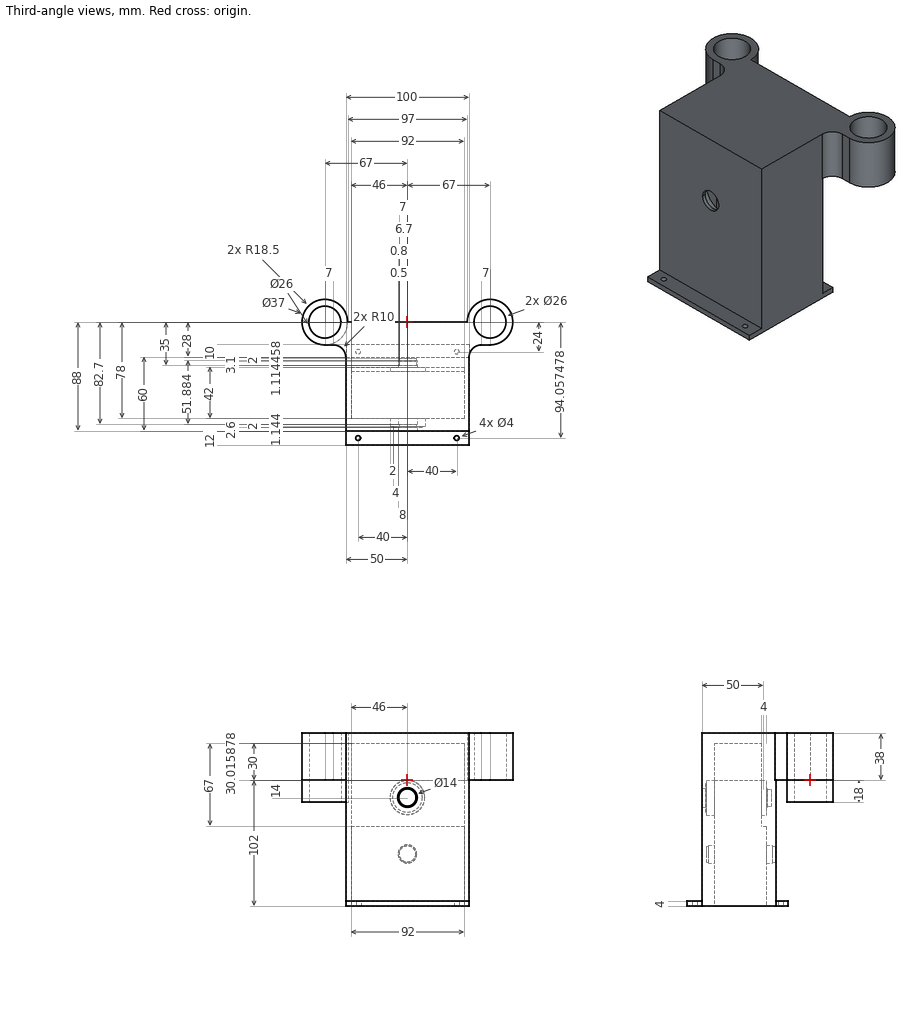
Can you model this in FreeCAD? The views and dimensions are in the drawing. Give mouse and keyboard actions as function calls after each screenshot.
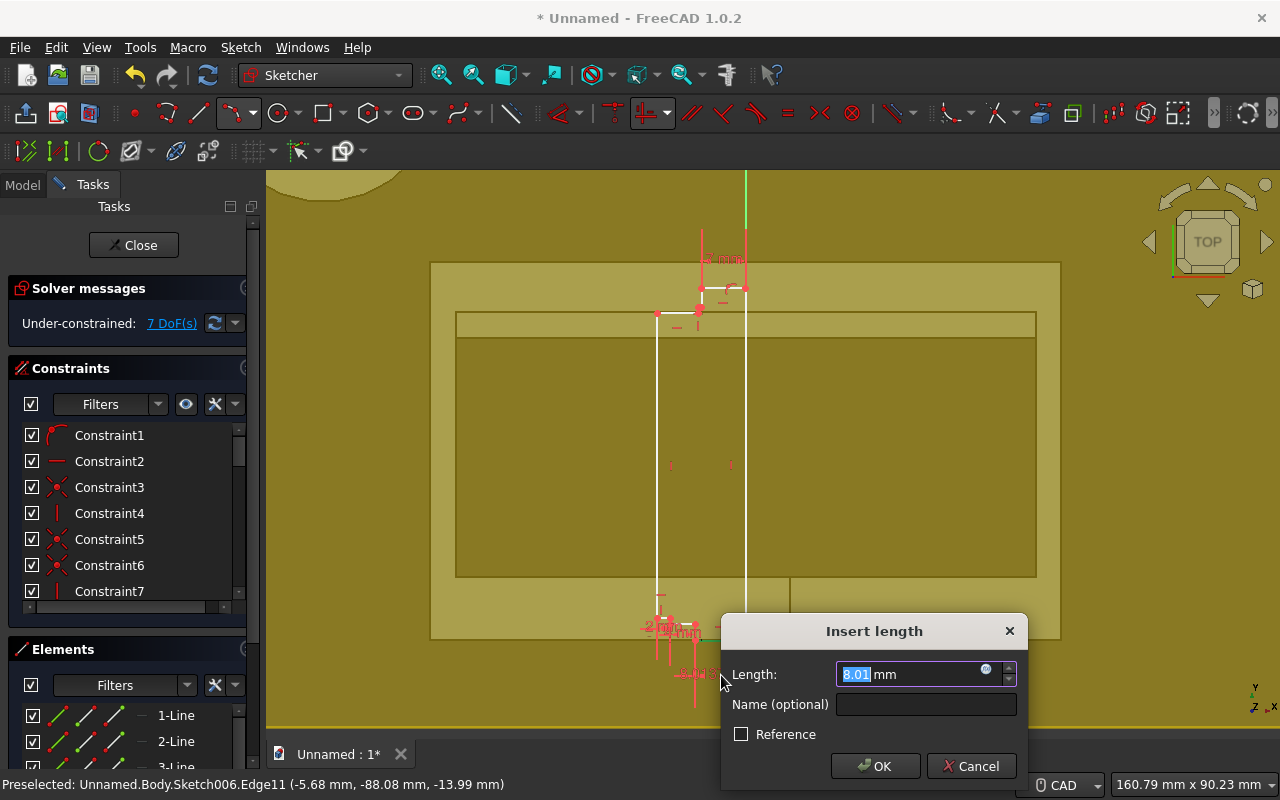
text(8)
key(Return)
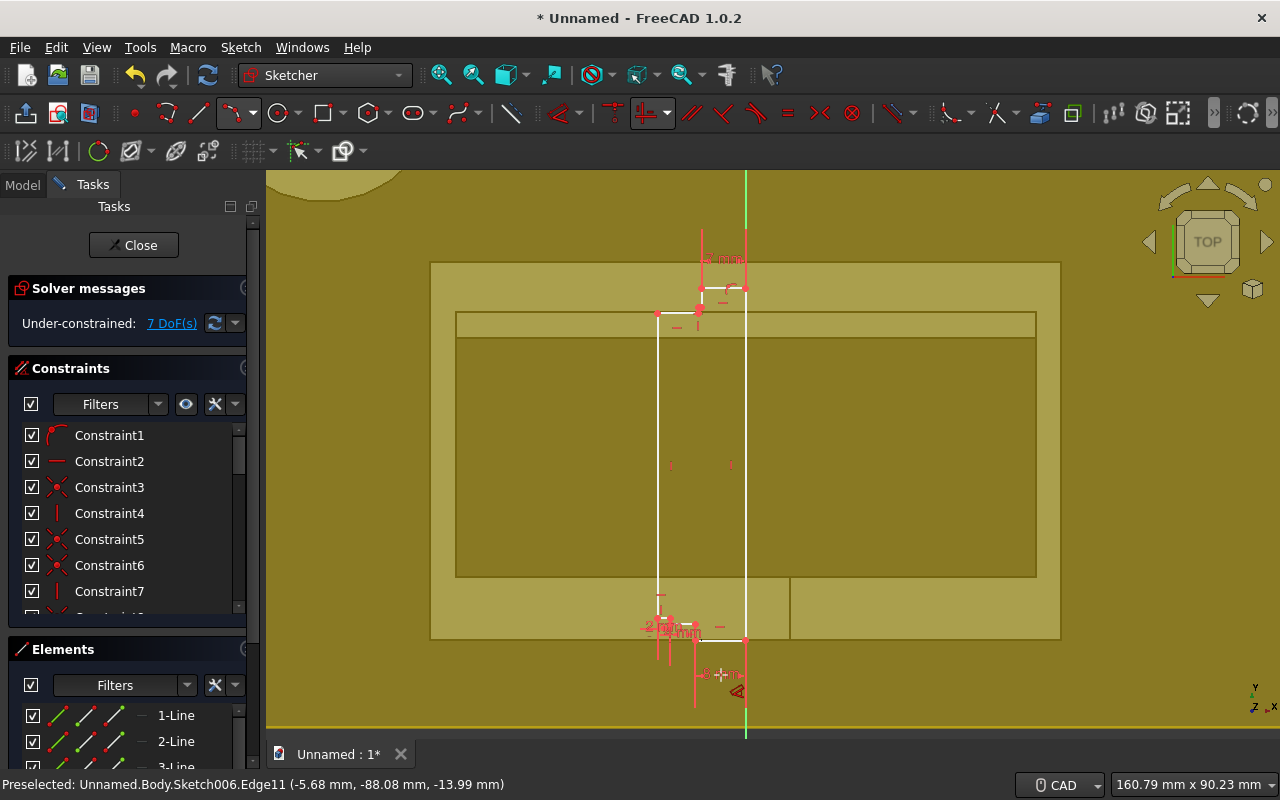
scroll(702, 298, up, 4)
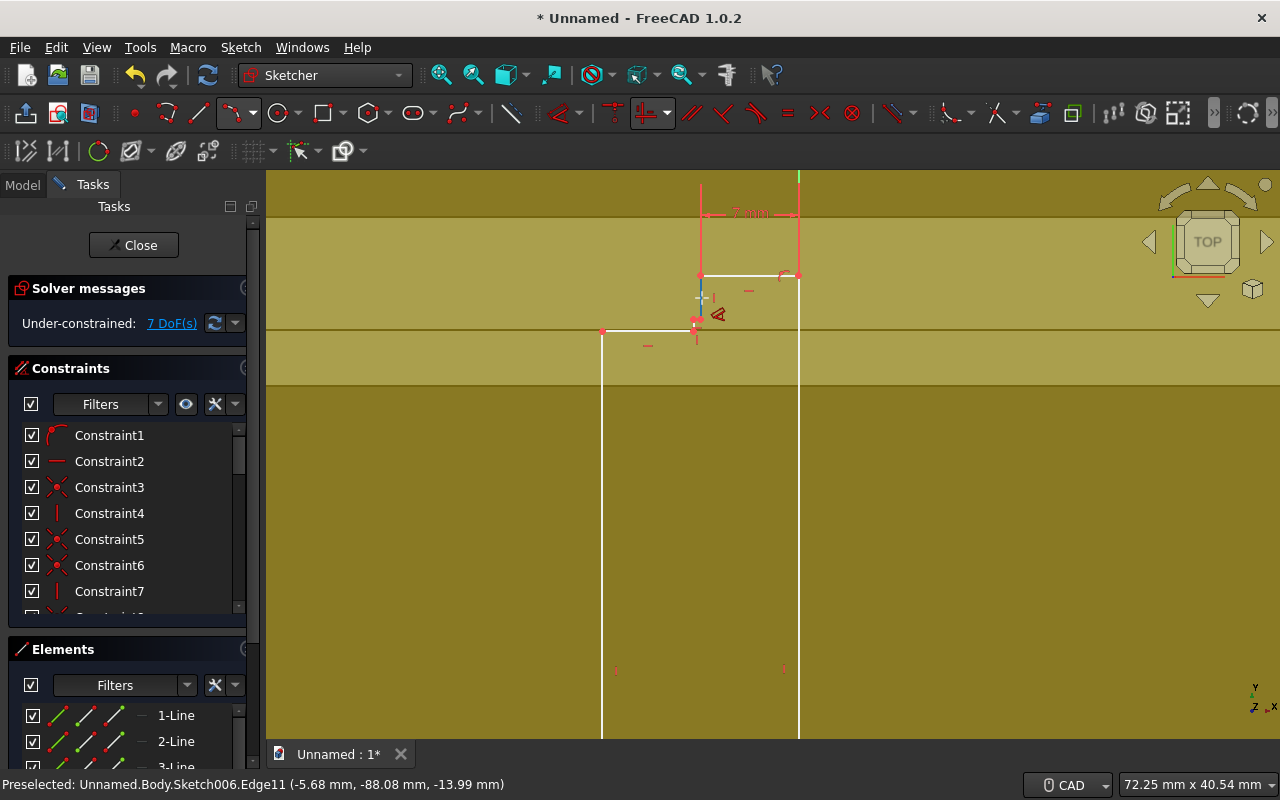
click(701, 298)
click(735, 298)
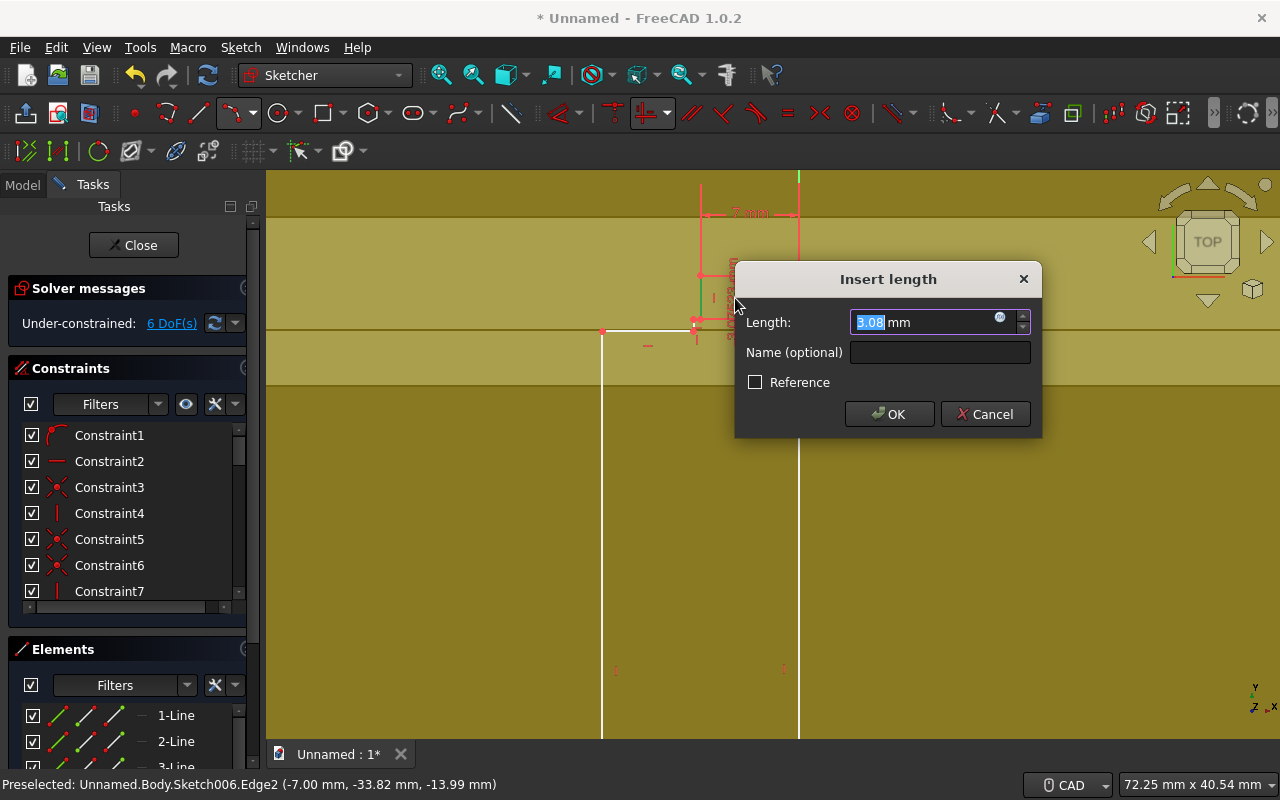
text(3.1)
key(Return)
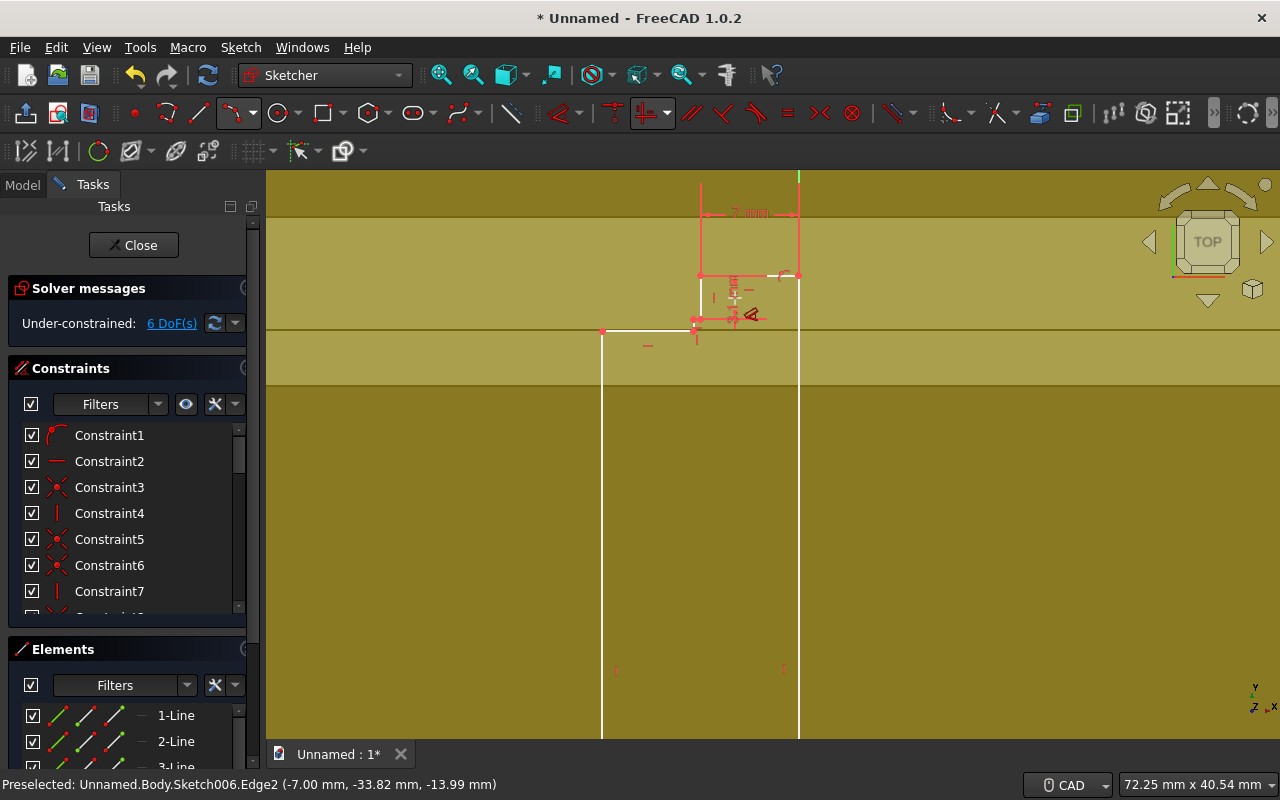
scroll(697, 319, up, 9)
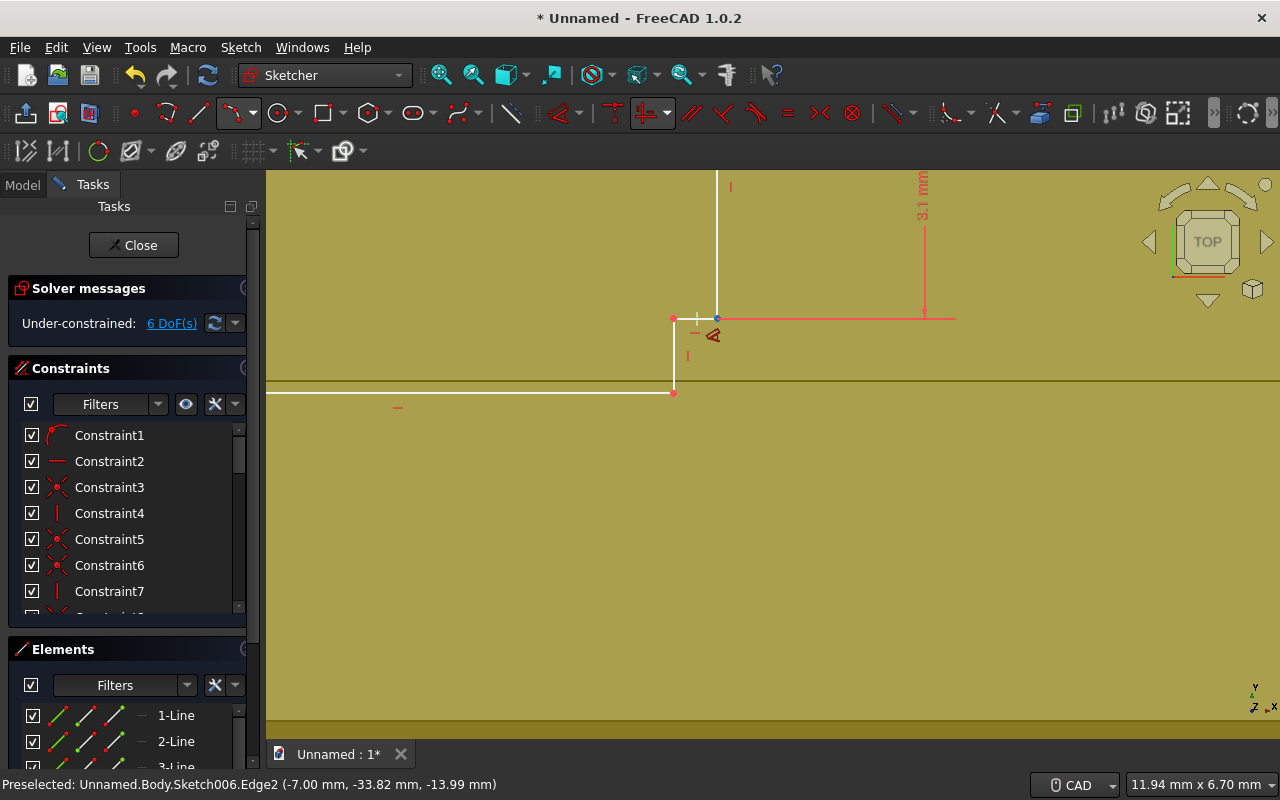
click(696, 319)
click(696, 285)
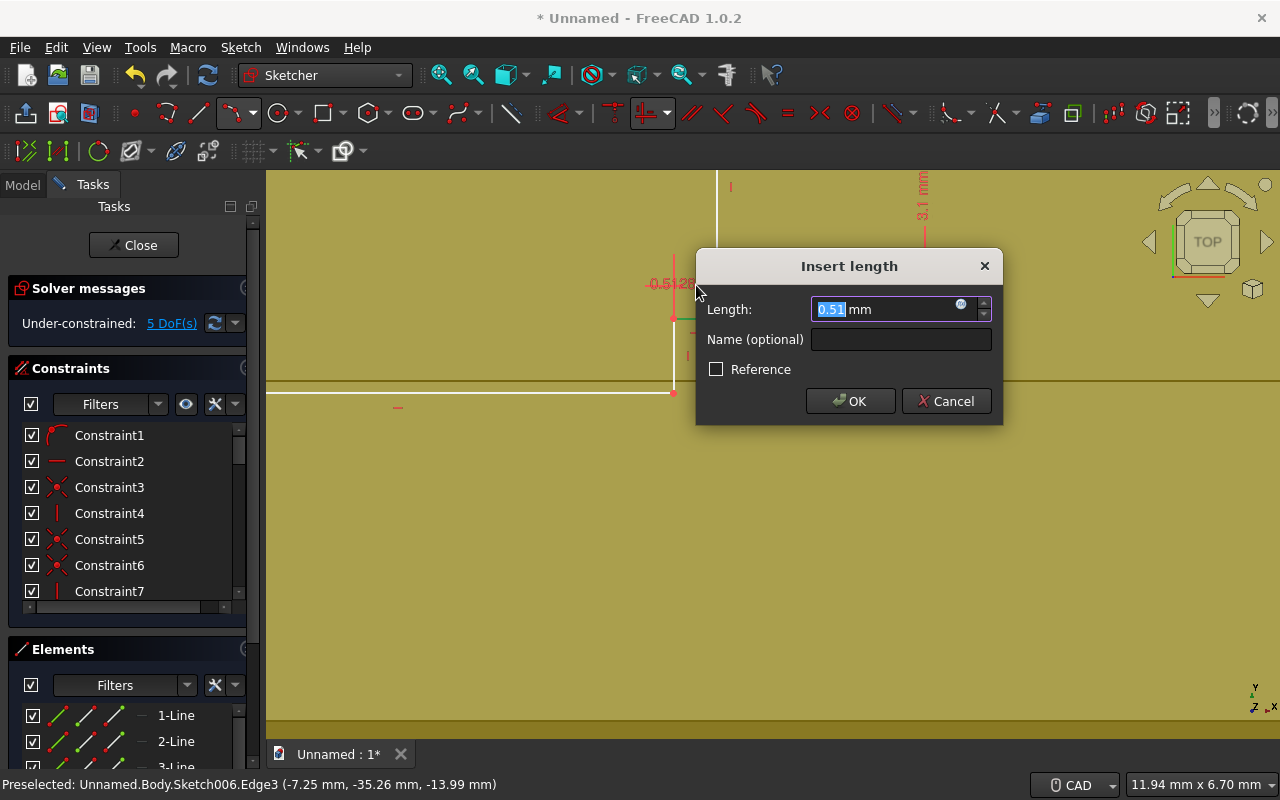
text(0.5)
key(Return)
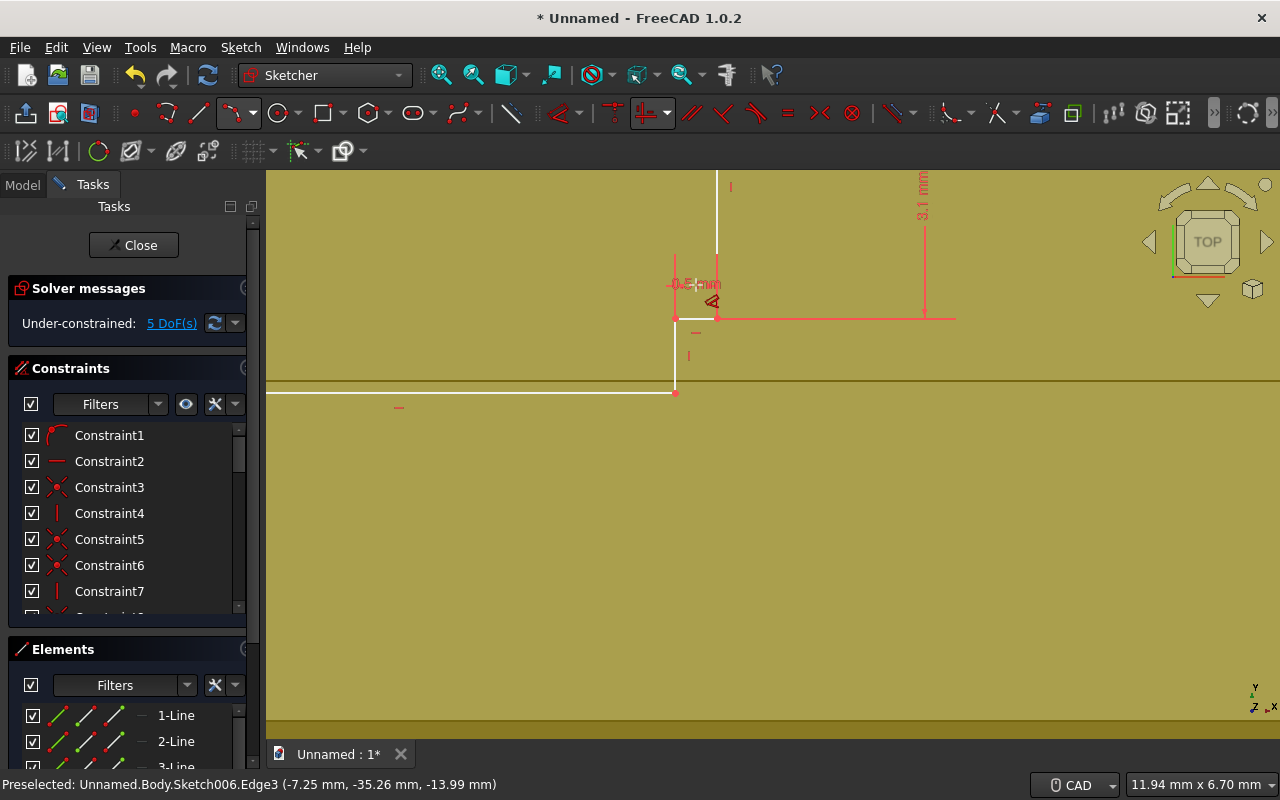
scroll(704, 423, down, 15)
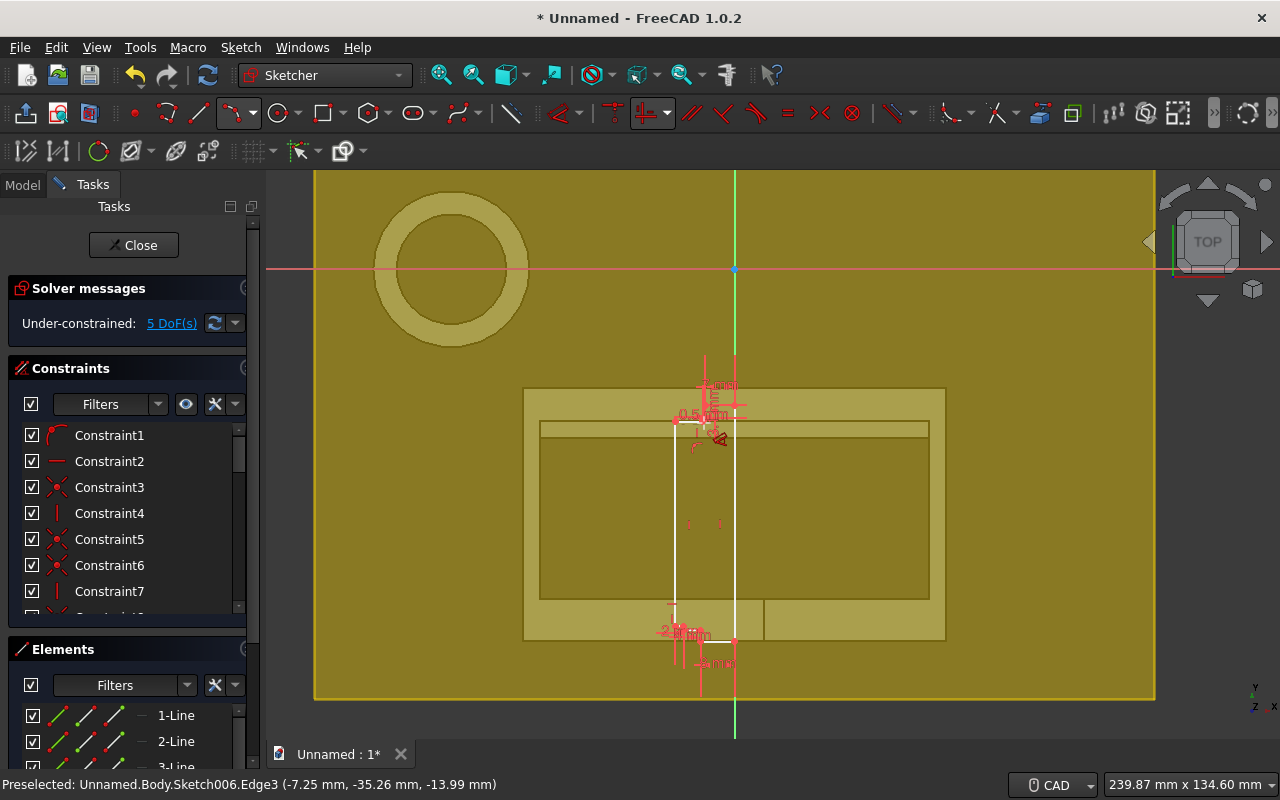
scroll(701, 634, up, 8)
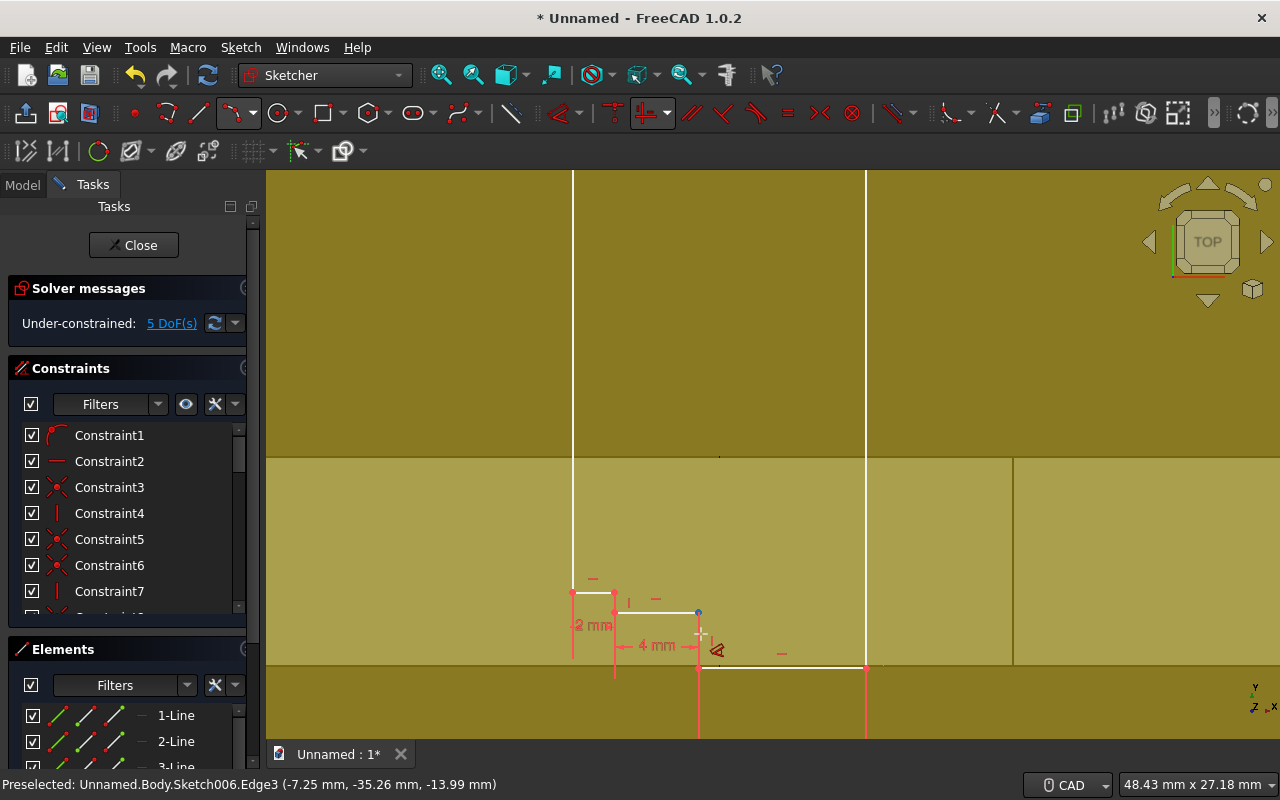
click(699, 629)
click(733, 640)